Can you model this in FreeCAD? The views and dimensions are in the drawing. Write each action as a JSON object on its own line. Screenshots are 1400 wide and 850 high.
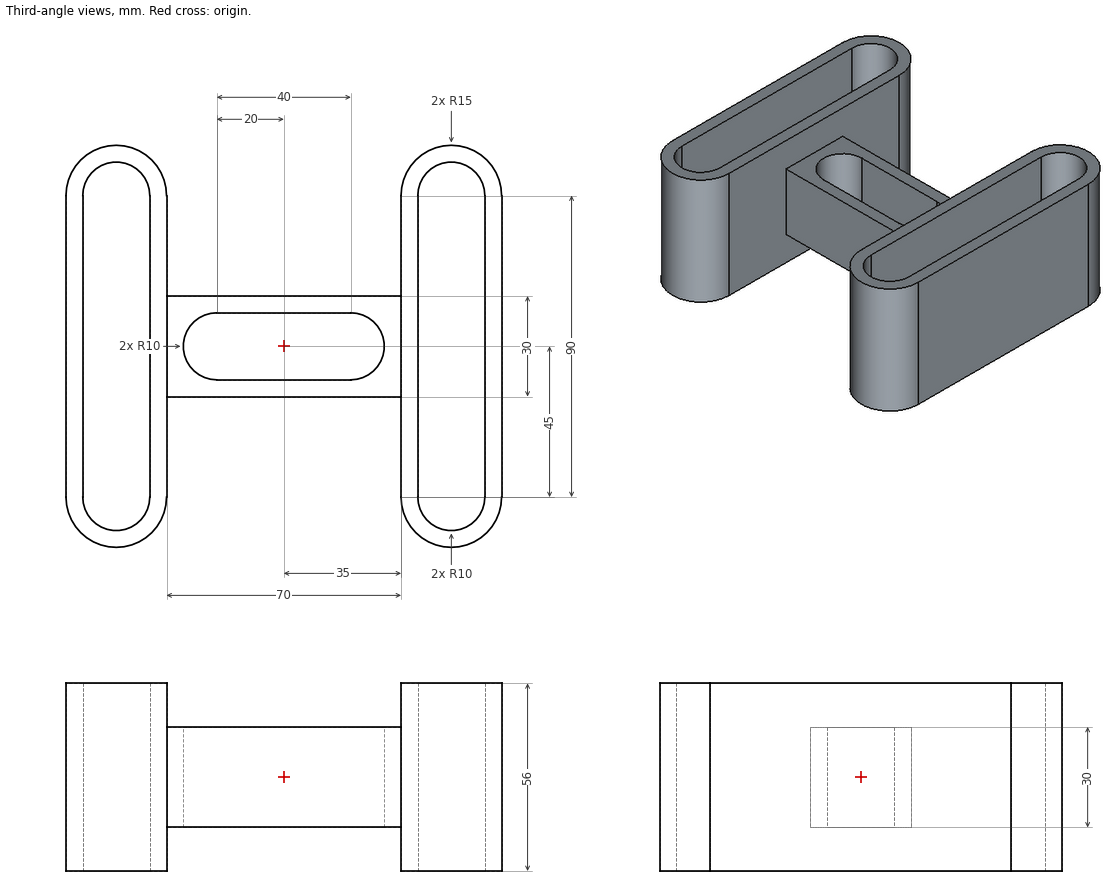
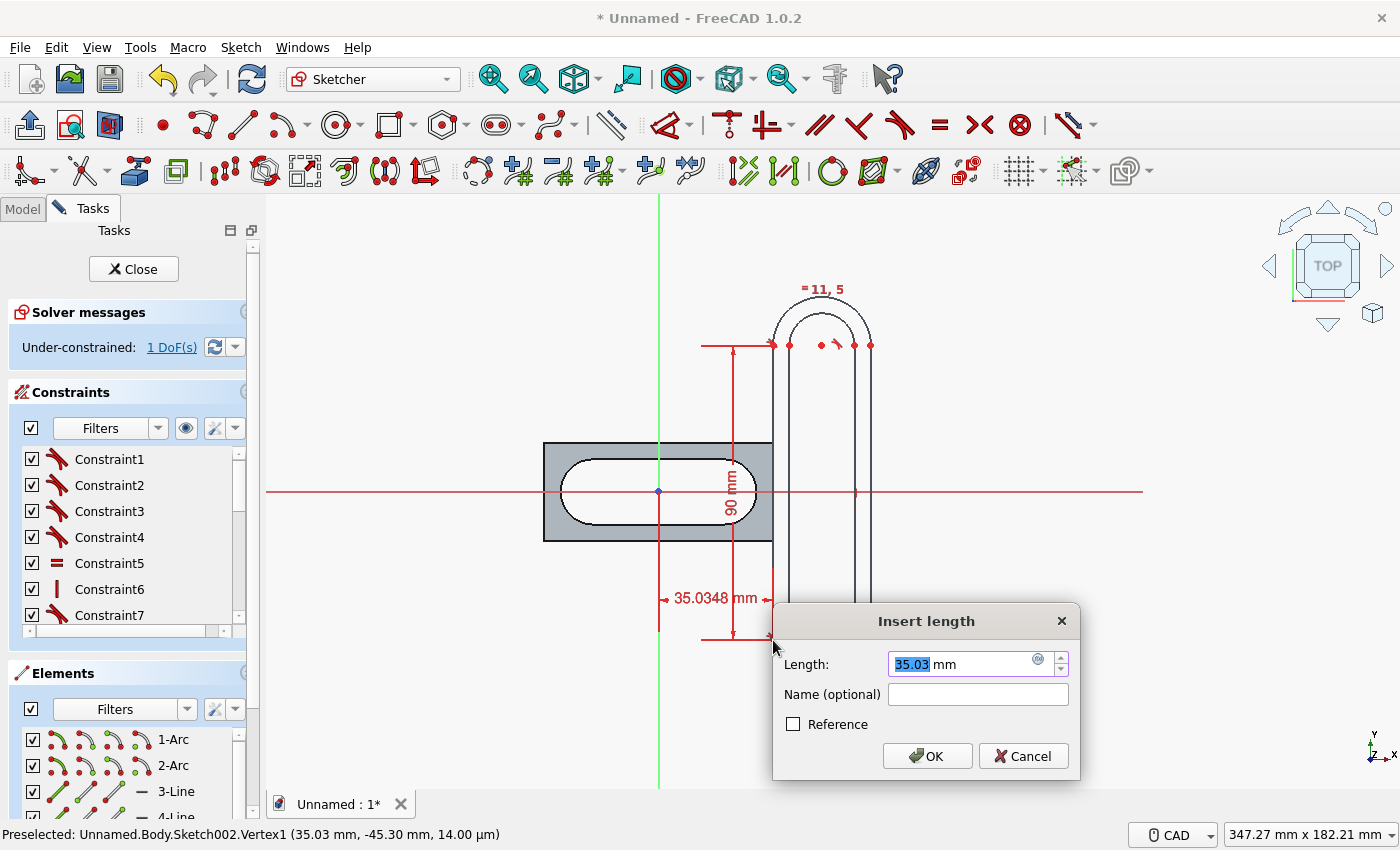
{"action": "type", "text": "35"}
{"action": "key", "text": "Return"}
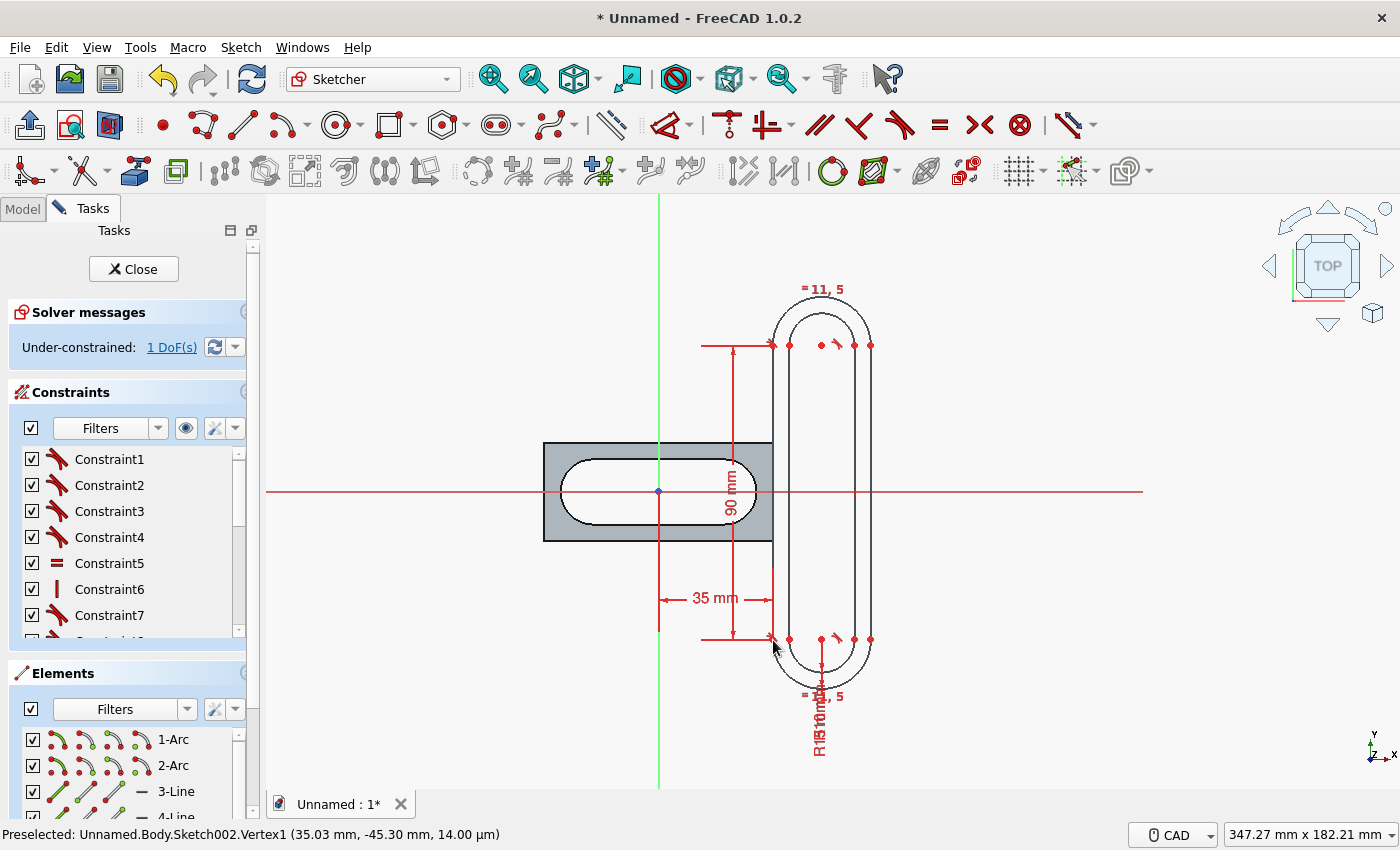
{"action": "left_click", "coordinate": [773, 640]}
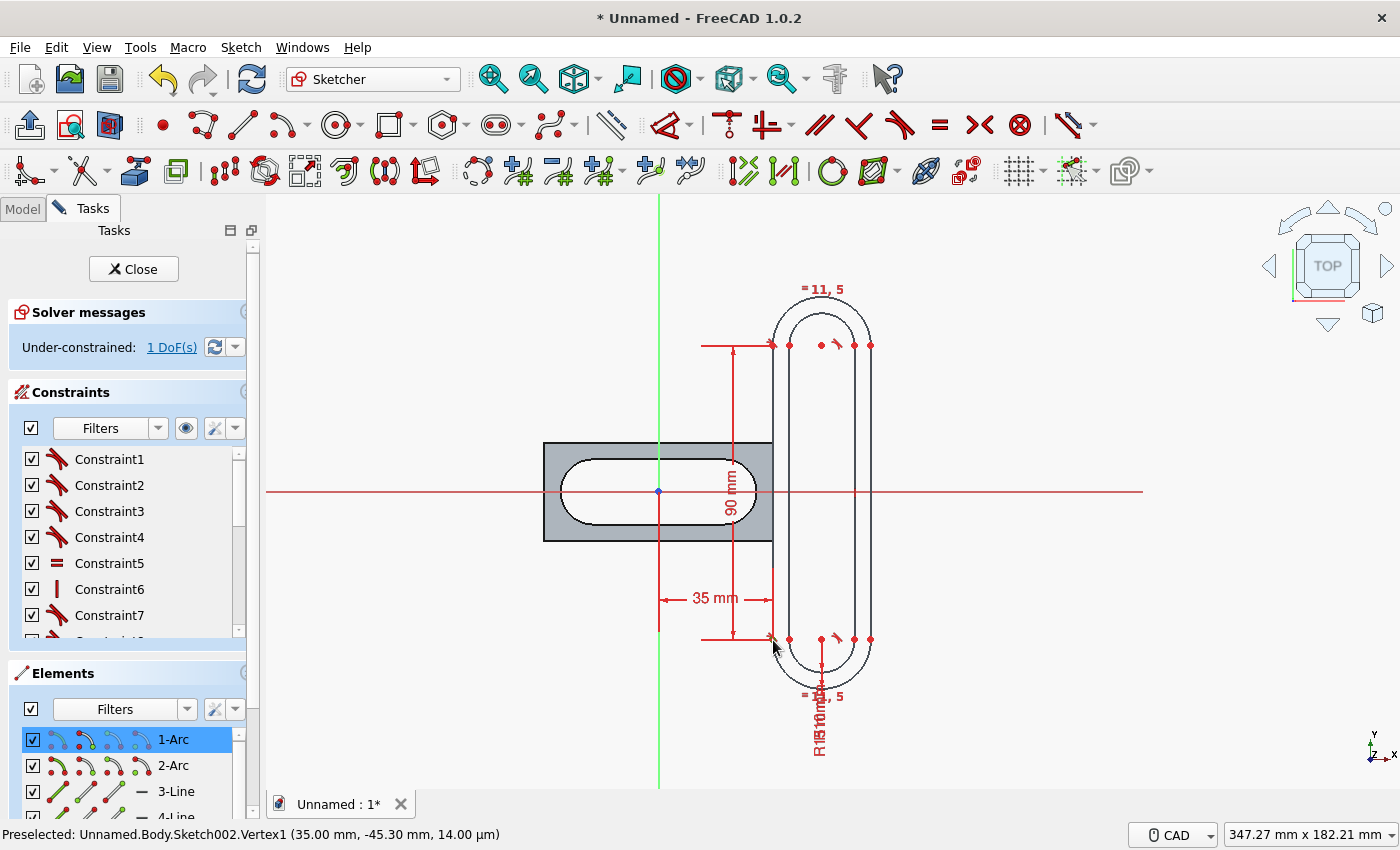
{"action": "left_click", "coordinate": [692, 126]}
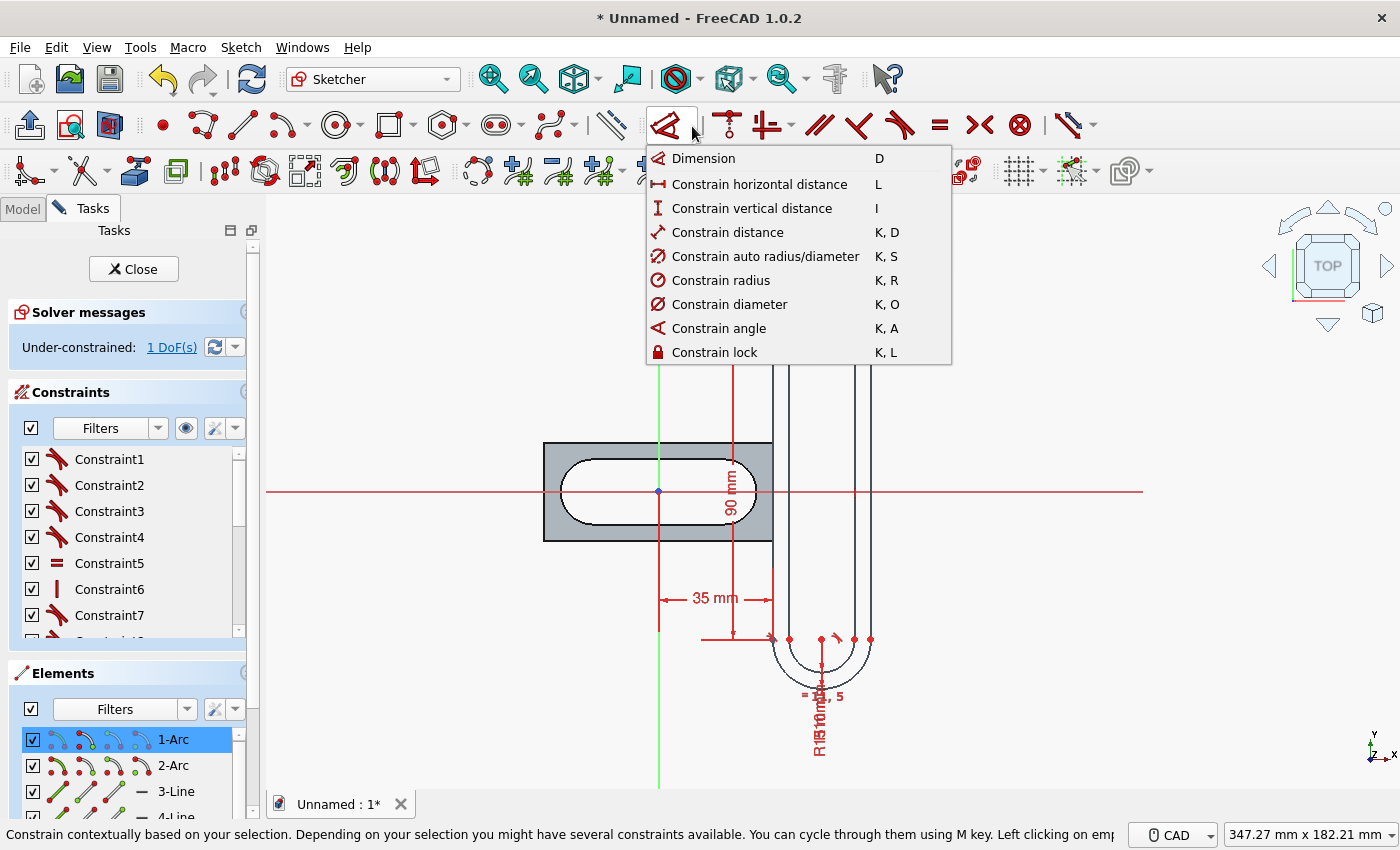
{"action": "left_click", "coordinate": [799, 208]}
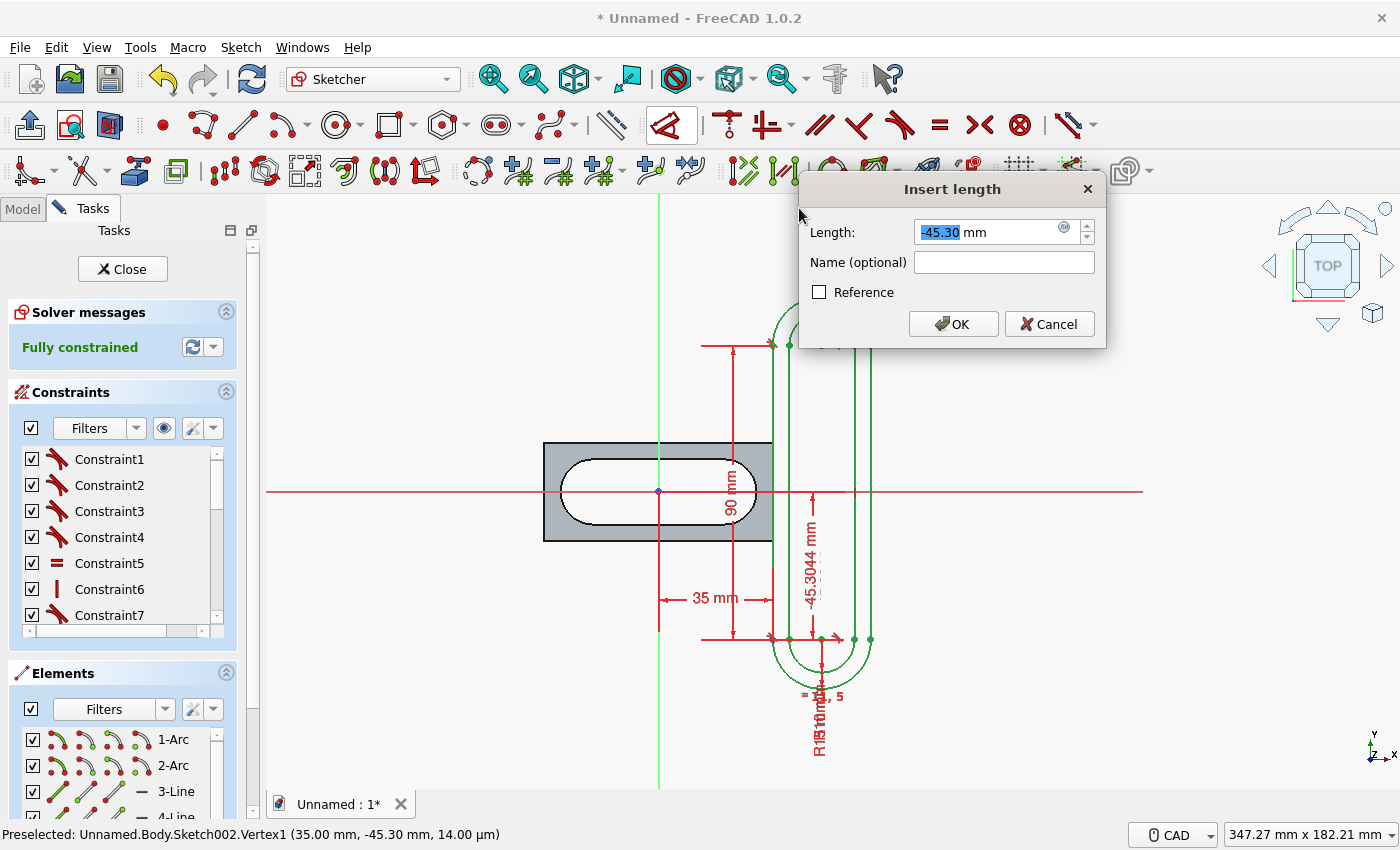
{"action": "type", "text": "-45"}
{"action": "key", "text": "Return"}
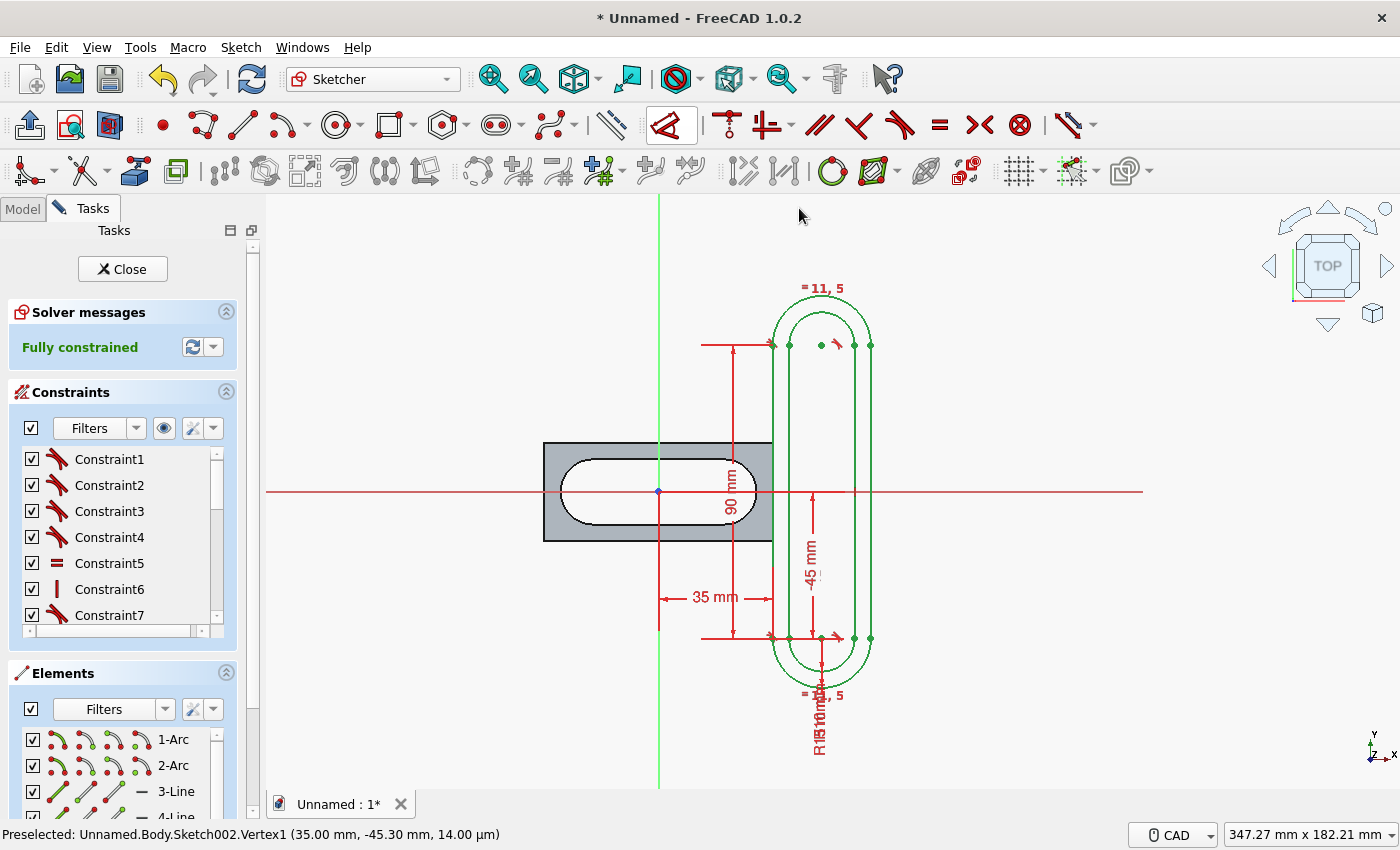
{"action": "left_click", "coordinate": [123, 269]}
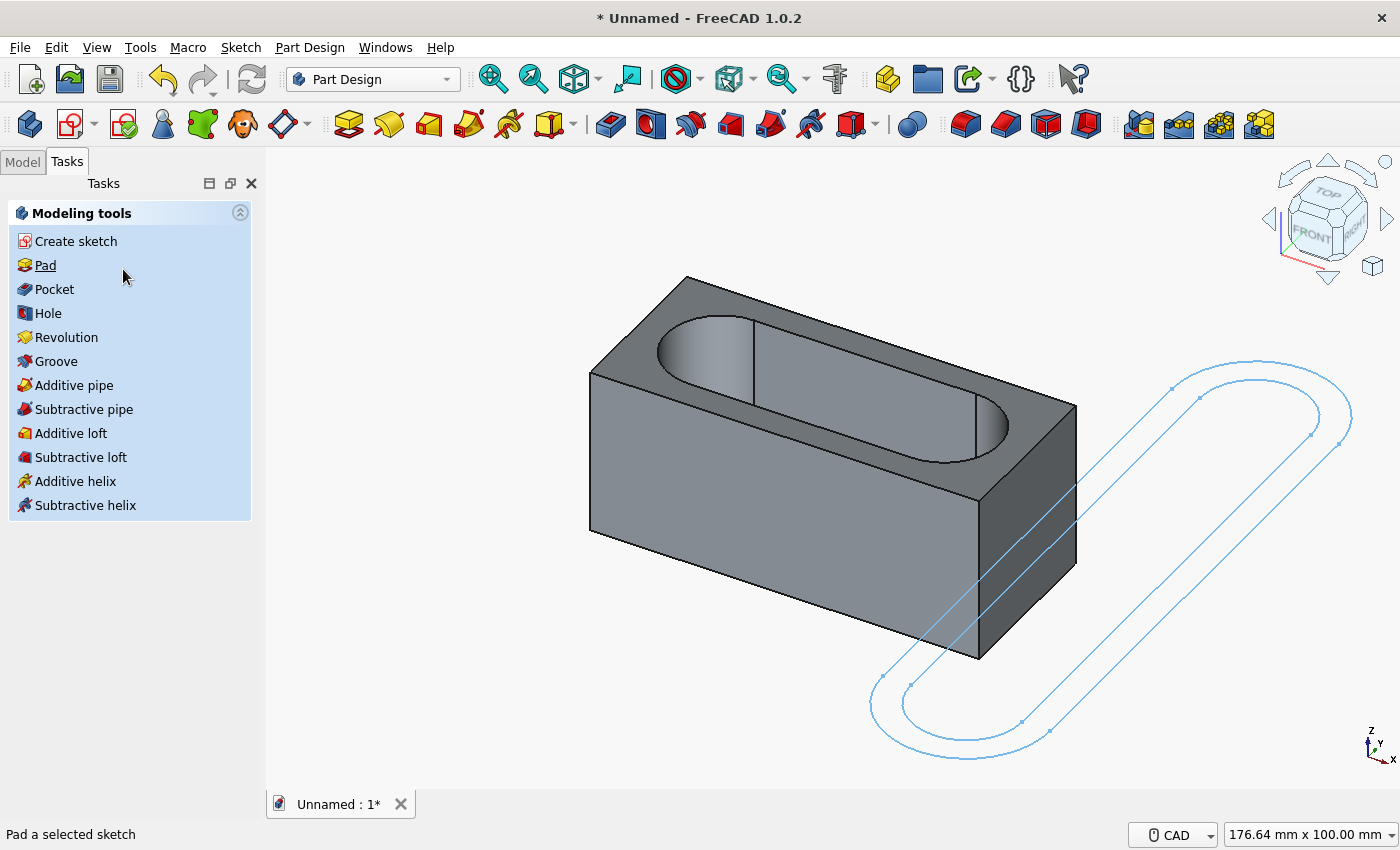
{"action": "left_click", "coordinate": [350, 124]}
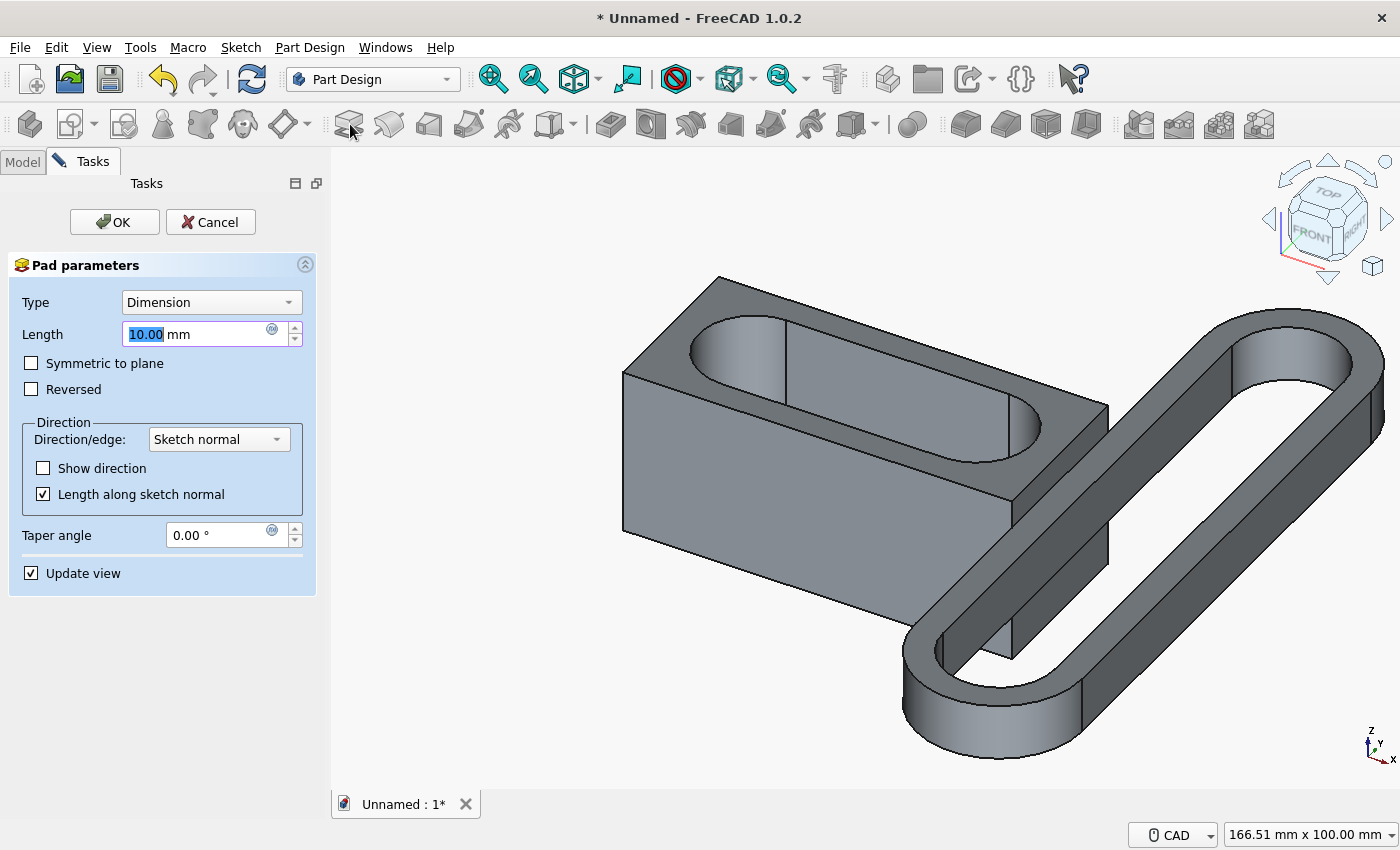
{"action": "type", "text": "56"}
{"action": "key", "text": "Tab"}